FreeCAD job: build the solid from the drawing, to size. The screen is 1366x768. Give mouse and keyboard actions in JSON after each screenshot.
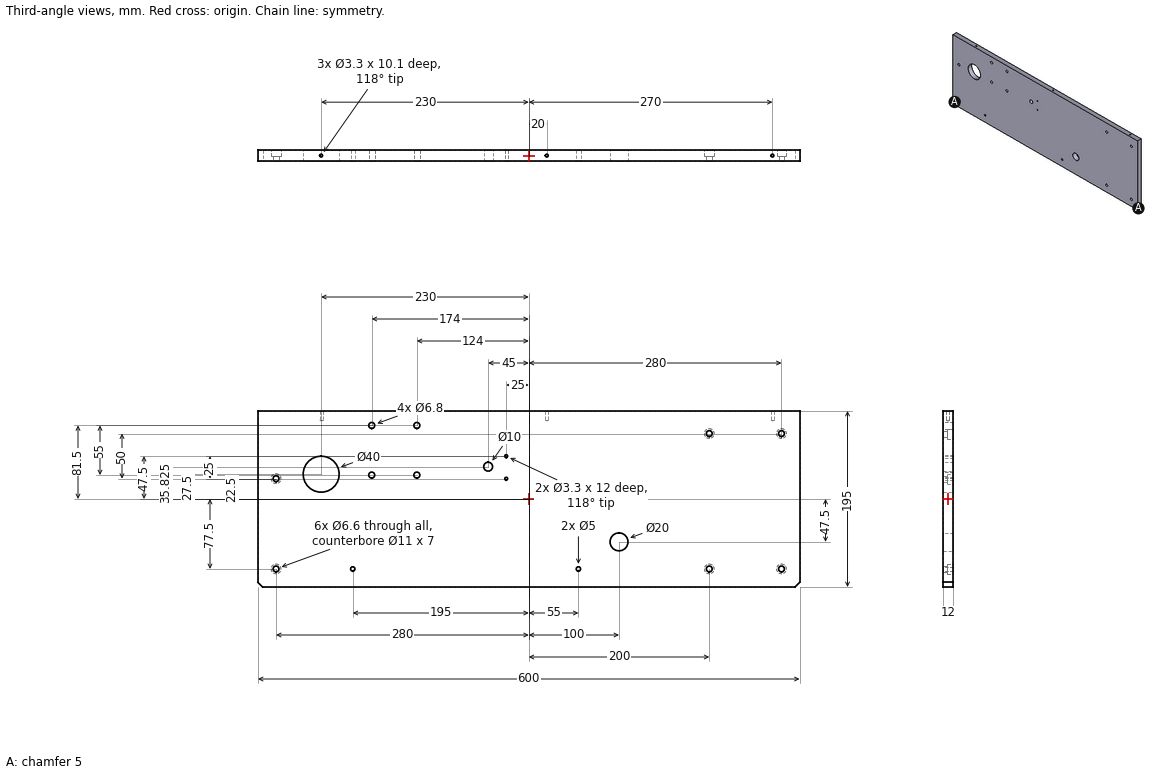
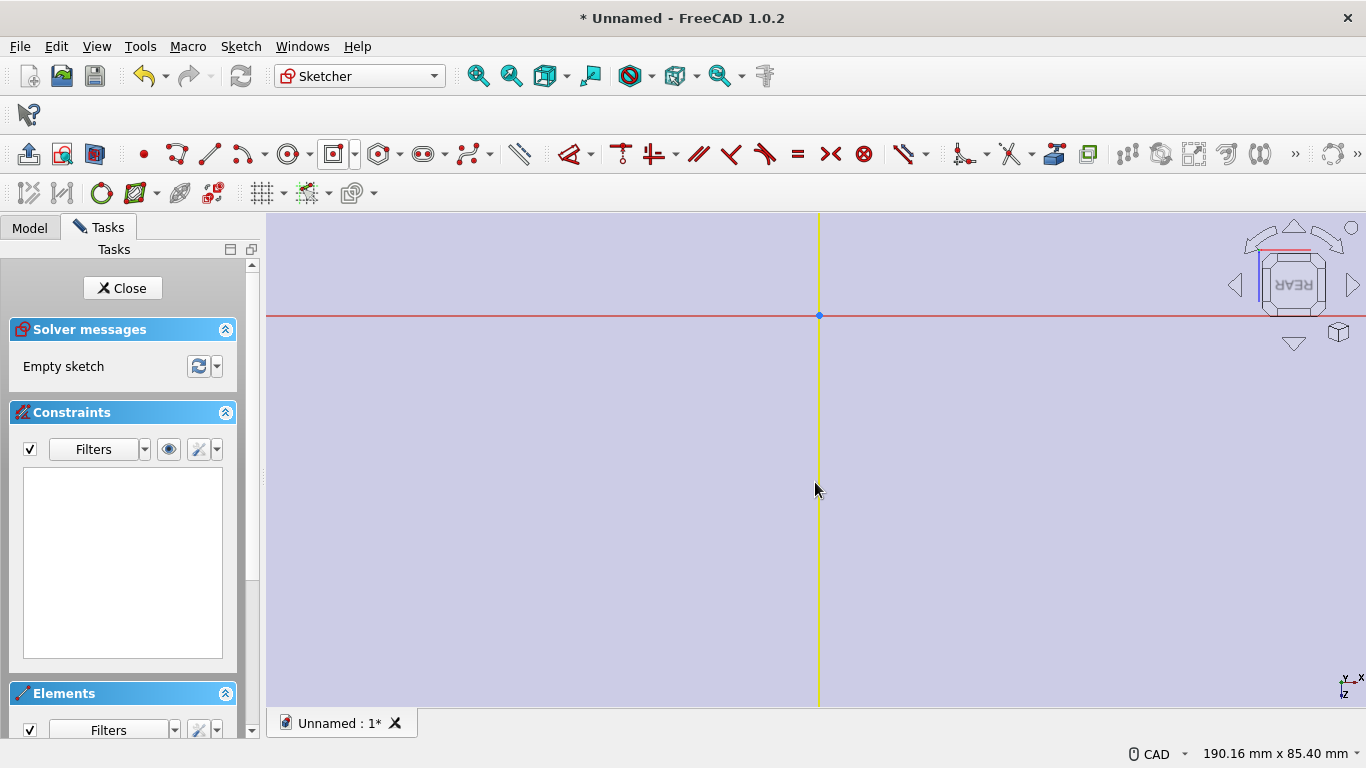
{"action": "key", "text": "g c"}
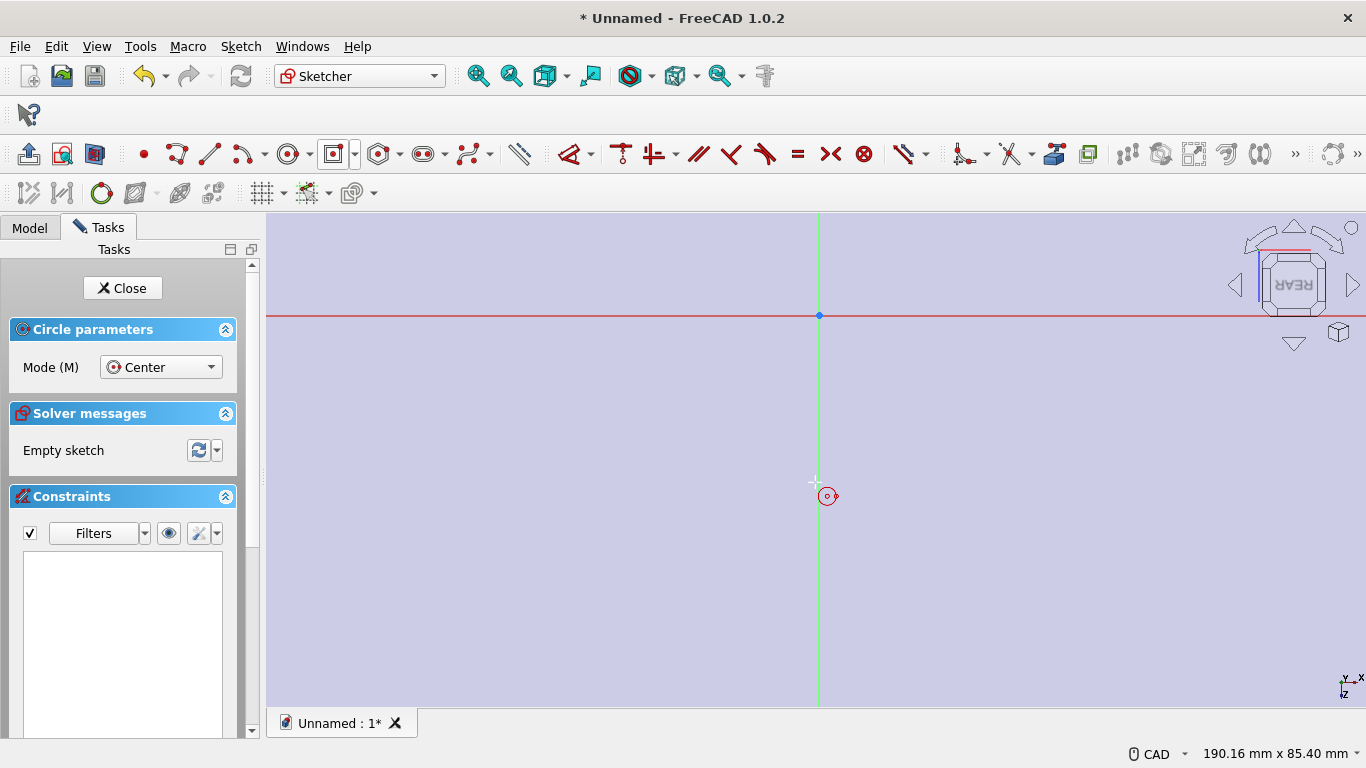
{"action": "scroll", "coordinate": [675, 591], "scroll_direction": "up", "scroll_amount": 5}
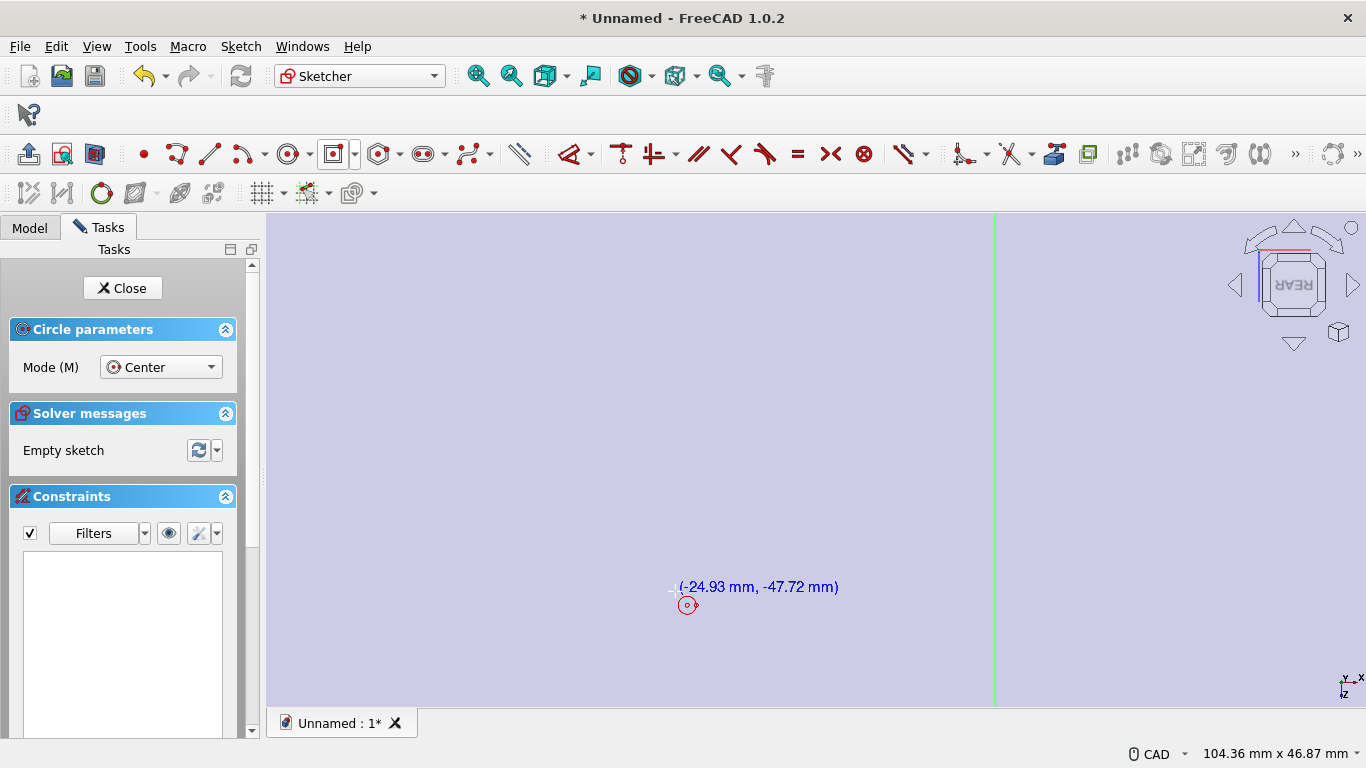
{"action": "left_click", "coordinate": [673, 589]}
{"action": "left_click", "coordinate": [692, 571]}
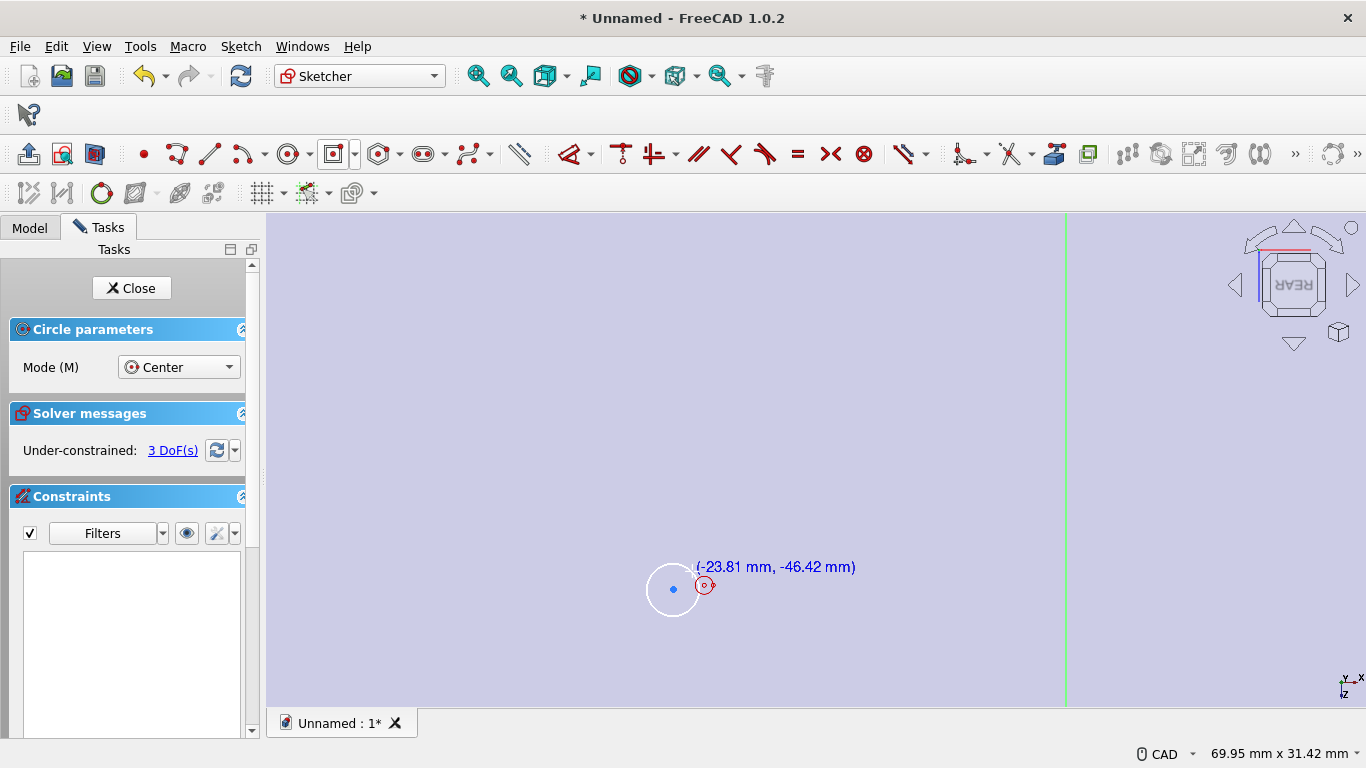
{"action": "scroll", "coordinate": [684, 595], "scroll_direction": "down", "scroll_amount": 5}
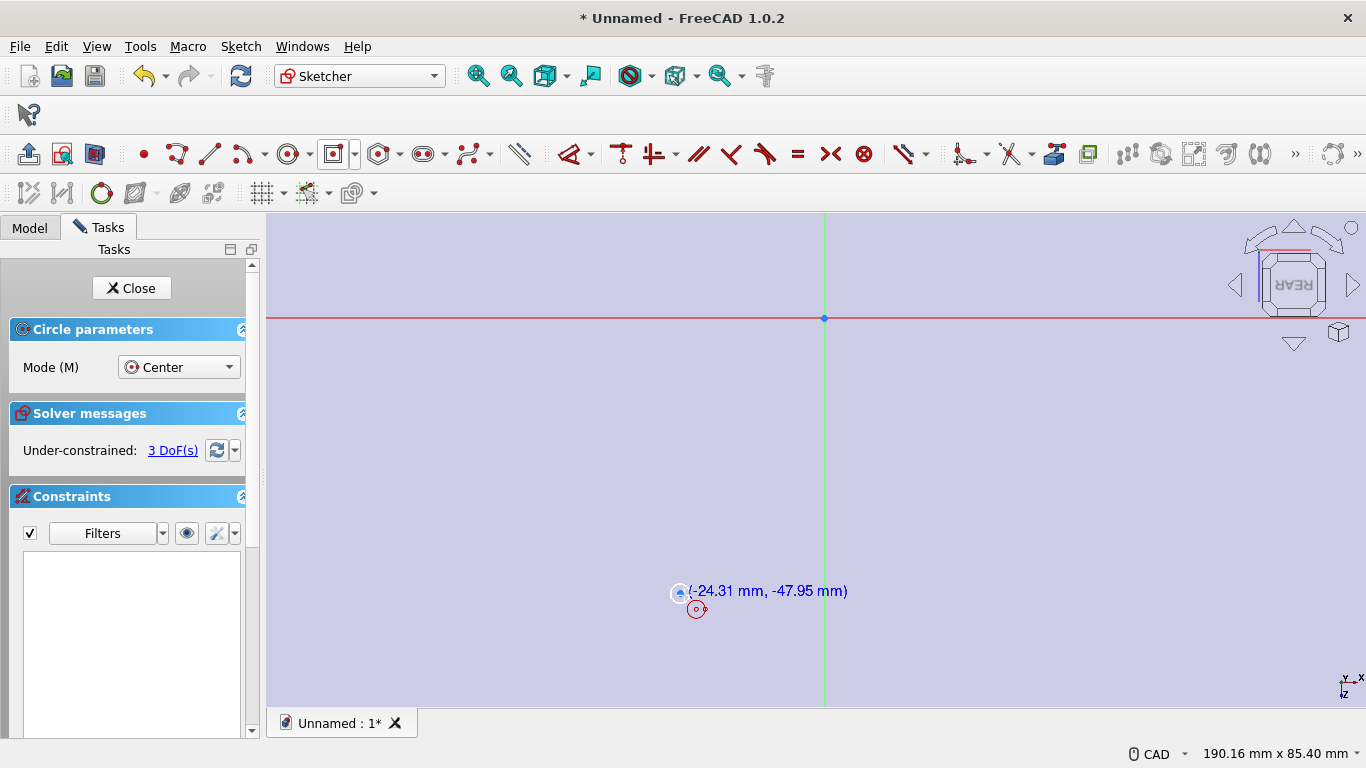
{"action": "scroll", "coordinate": [680, 449], "scroll_direction": "up", "scroll_amount": 5}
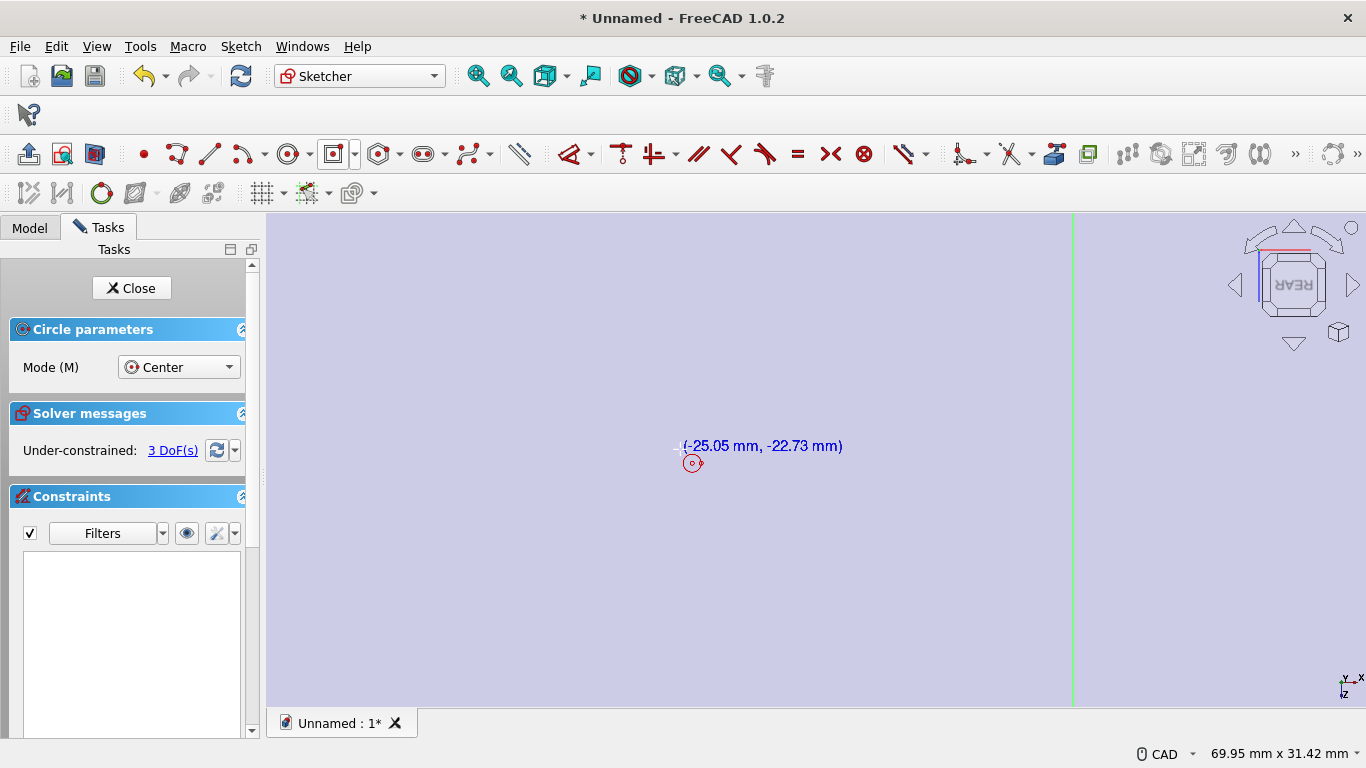
{"action": "left_click", "coordinate": [680, 447]}
{"action": "left_click", "coordinate": [698, 429]}
{"action": "key", "text": "Escape"}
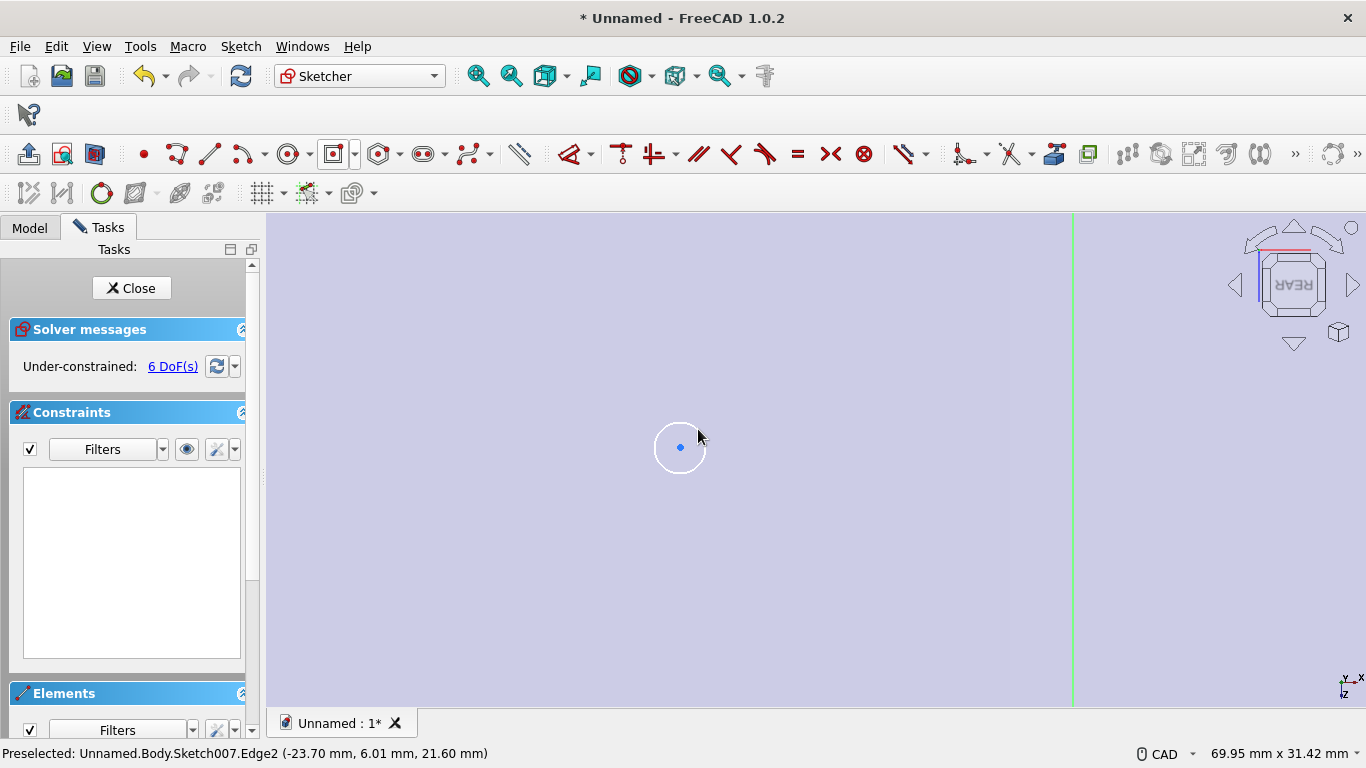
{"action": "scroll", "coordinate": [680, 448], "scroll_direction": "down", "scroll_amount": 5}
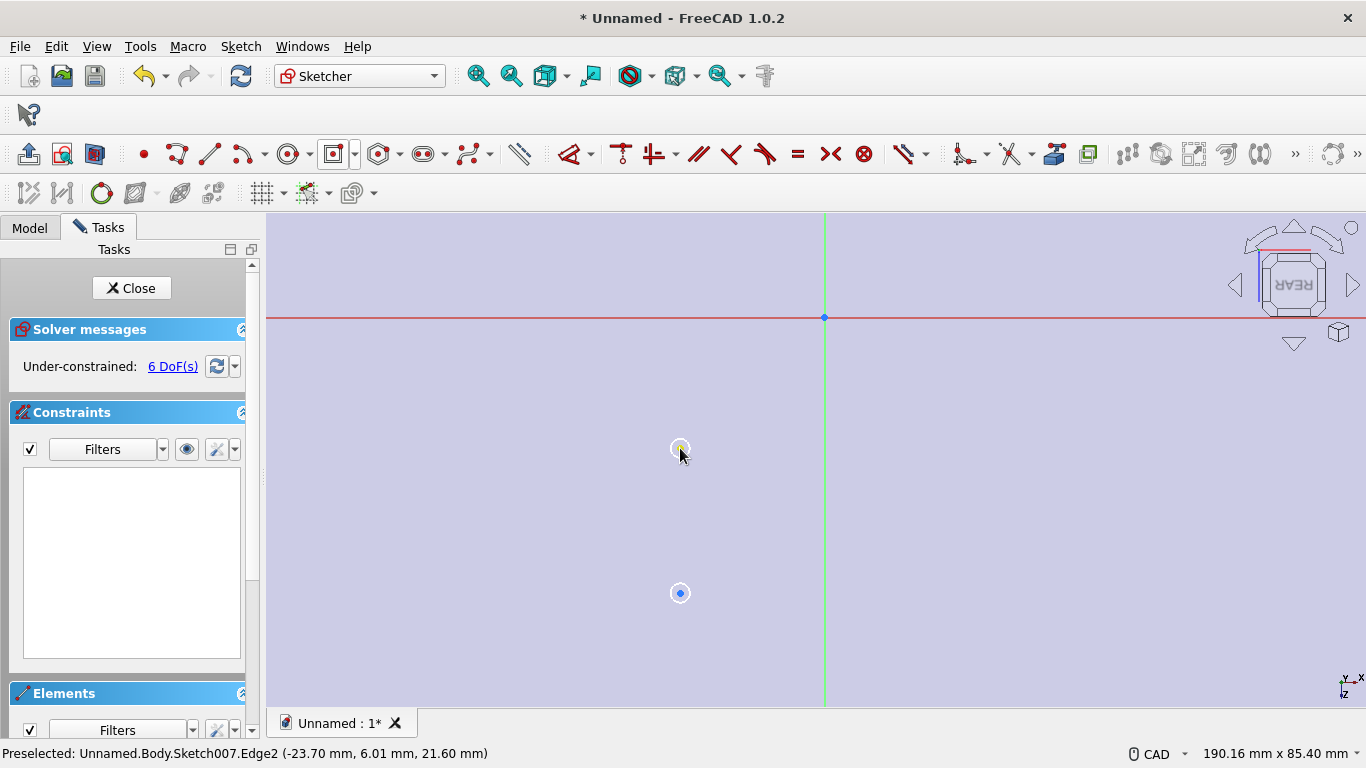
{"action": "scroll", "coordinate": [687, 586], "scroll_direction": "up", "scroll_amount": 2}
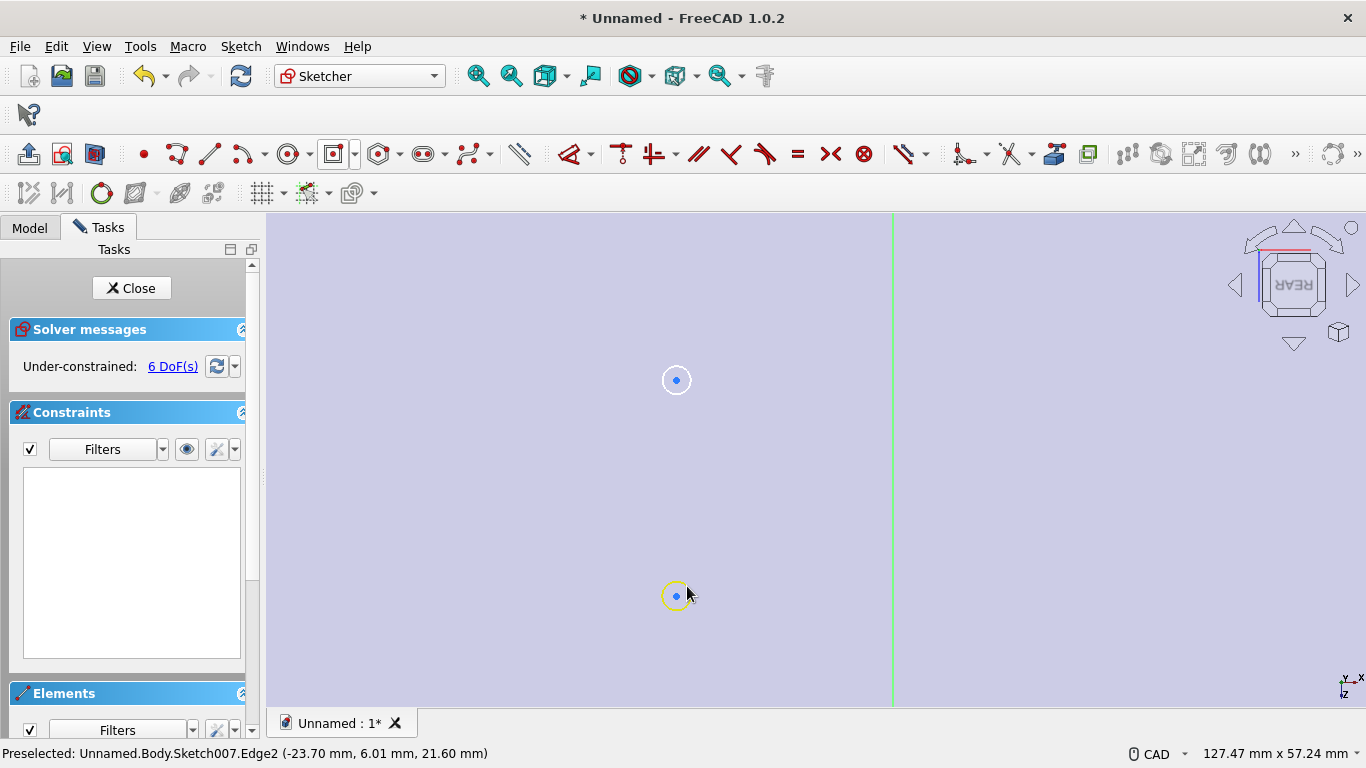
{"action": "left_click", "coordinate": [687, 586]}